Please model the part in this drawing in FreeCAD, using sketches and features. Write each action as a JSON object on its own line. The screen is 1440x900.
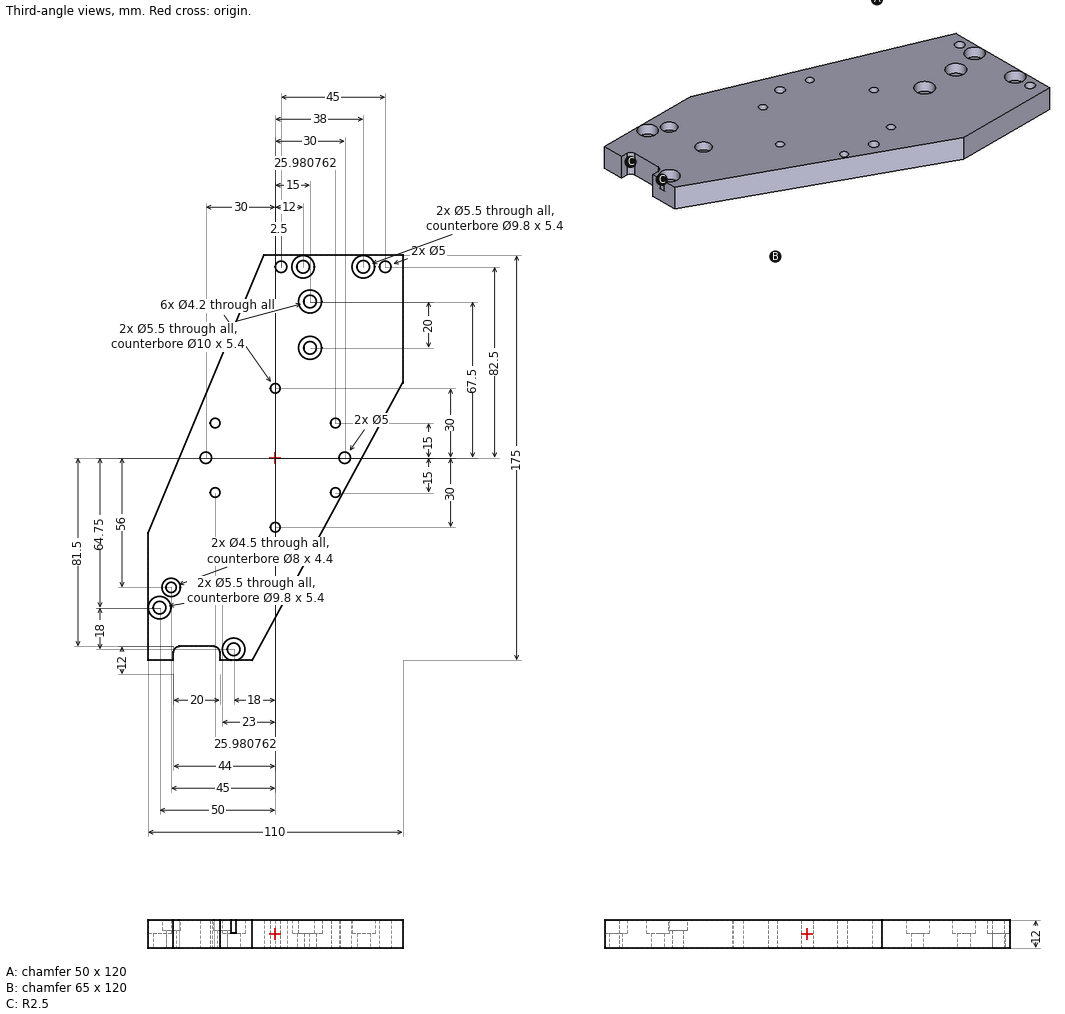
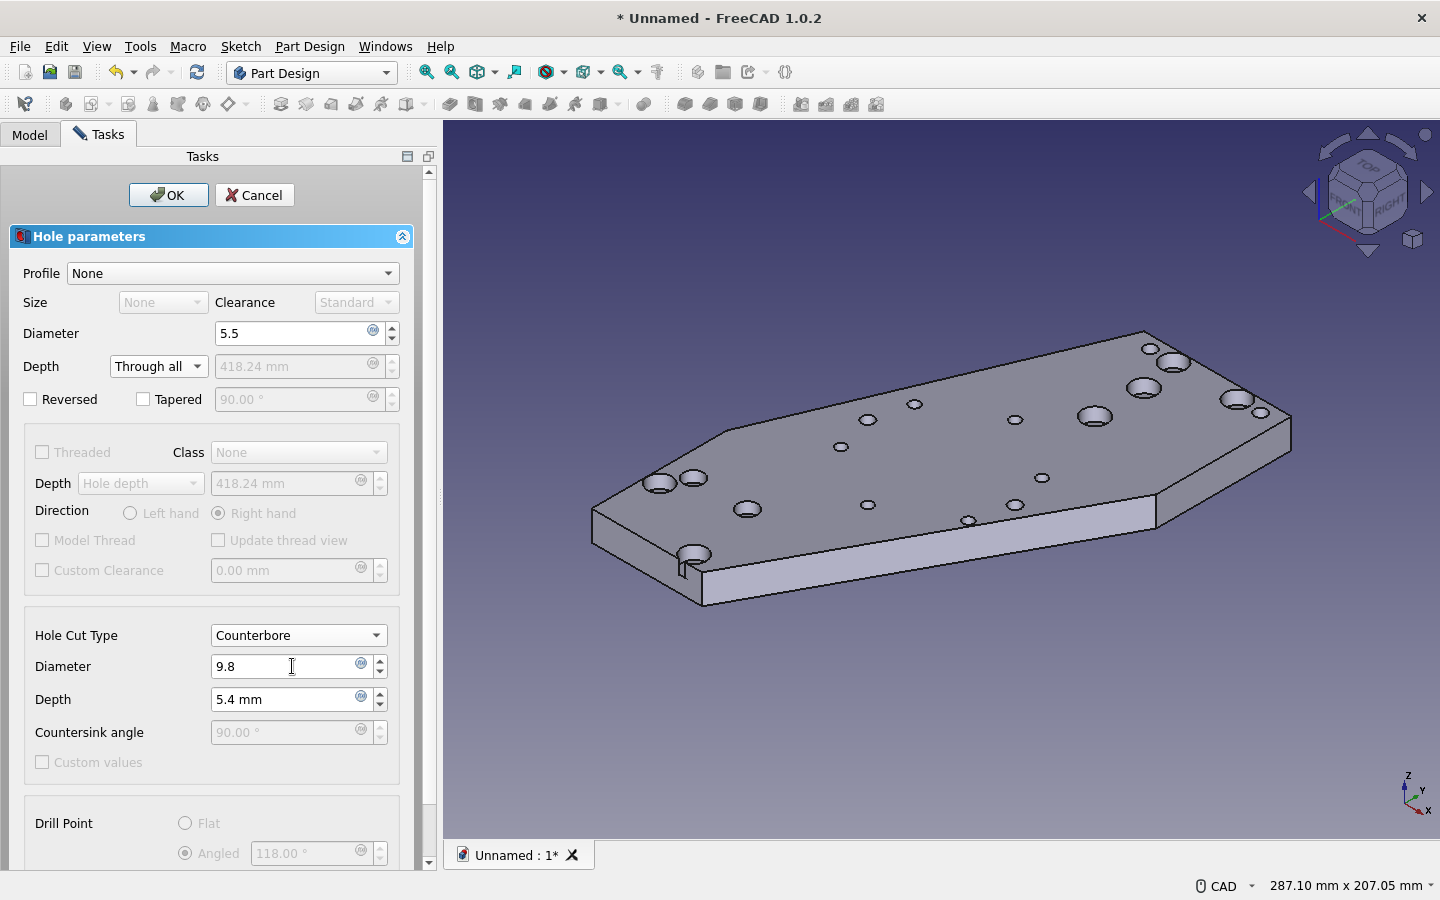
{"action": "left_click", "coordinate": [169, 195]}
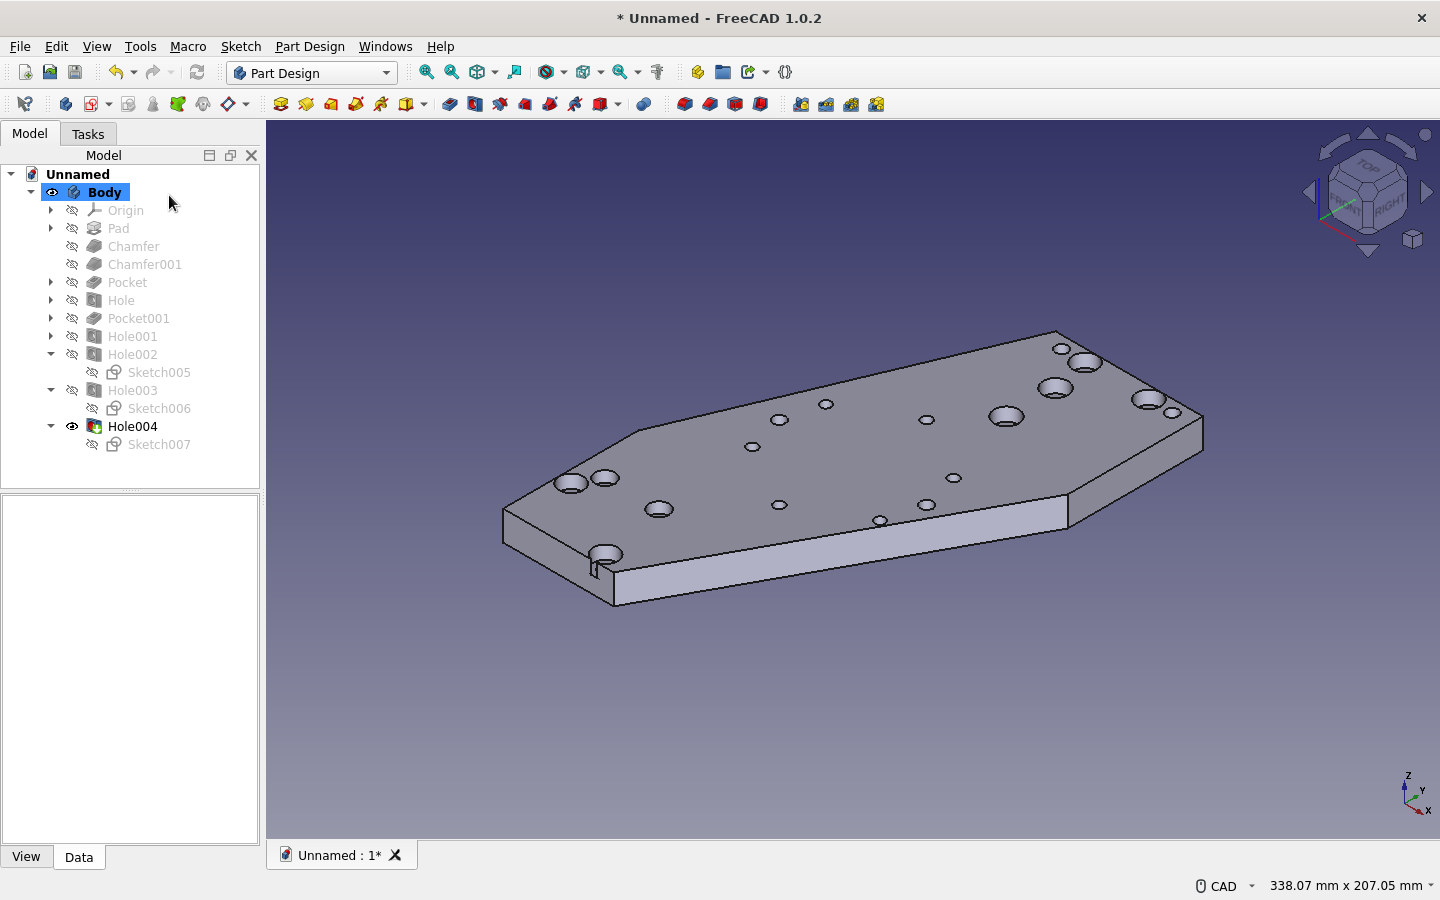
{"action": "left_click", "coordinate": [853, 461]}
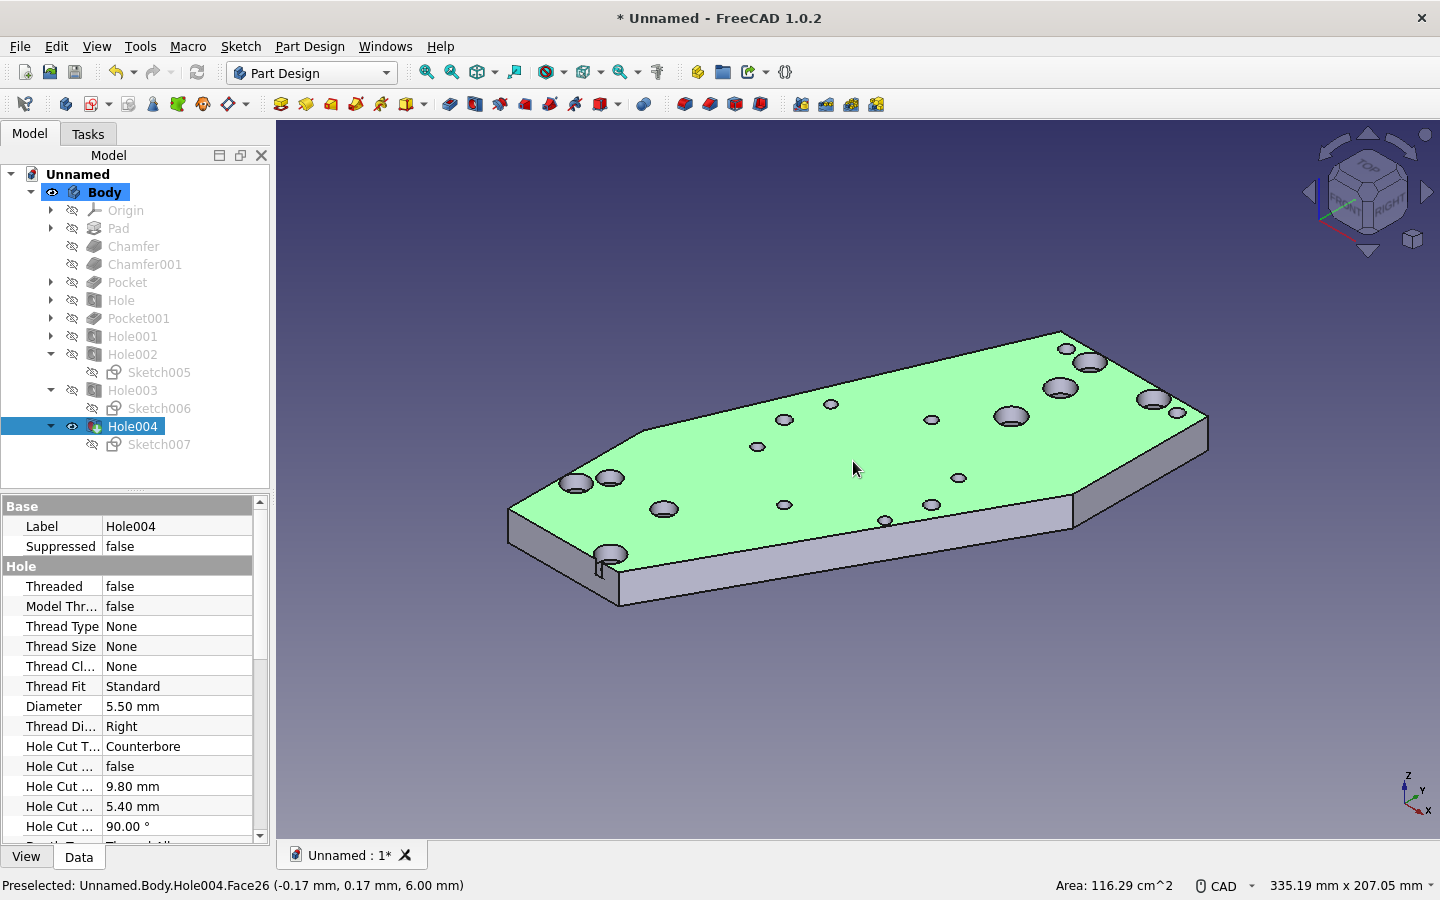
{"action": "left_click", "coordinate": [90, 104]}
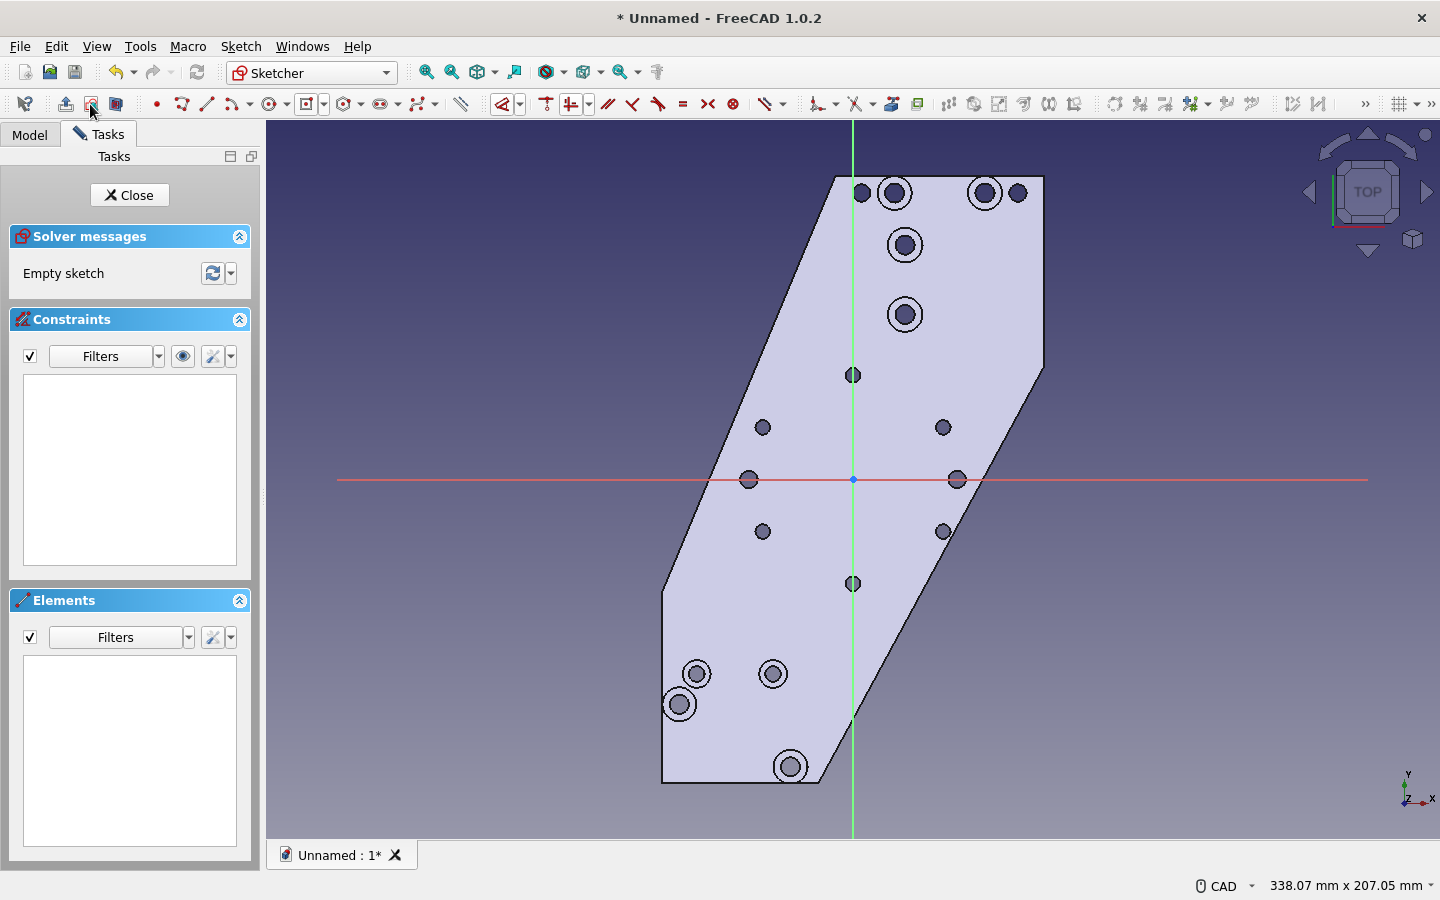
{"action": "scroll", "coordinate": [729, 811], "scroll_direction": "up", "scroll_amount": 11}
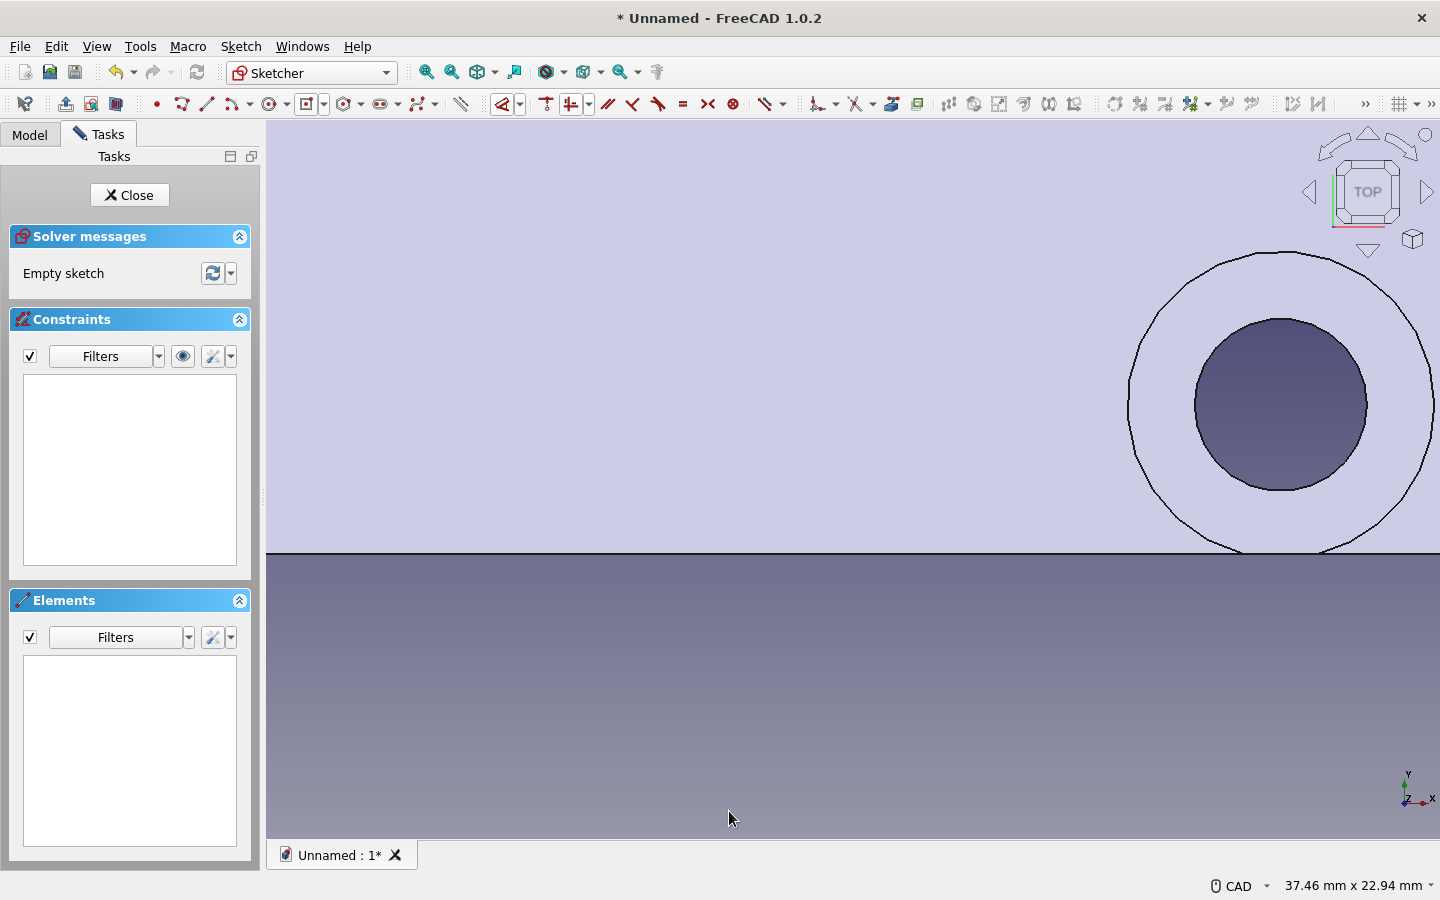
{"action": "key", "text": "g r"}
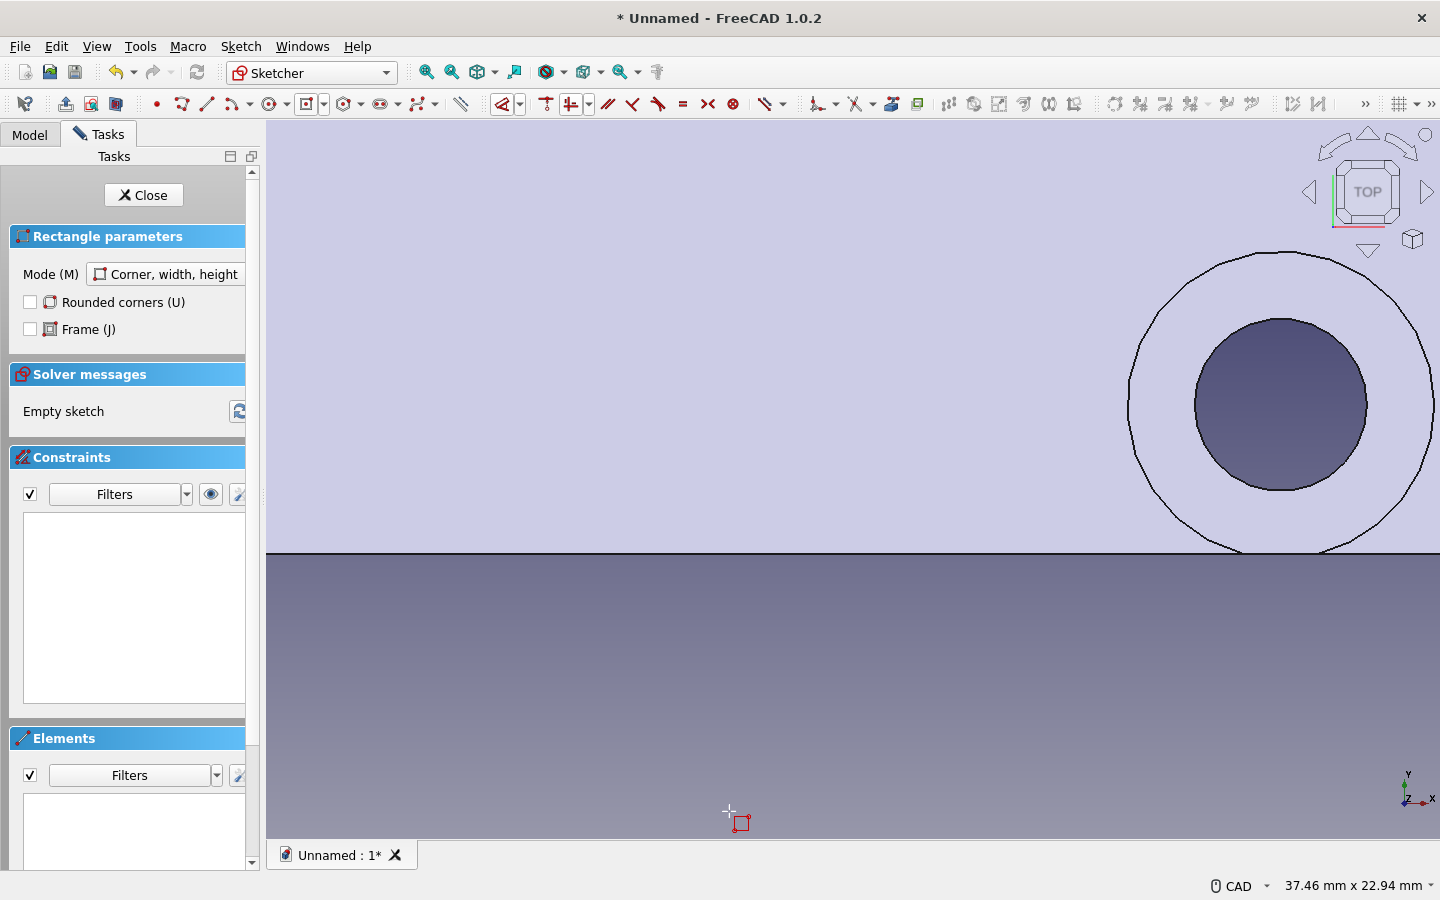
{"action": "left_click", "coordinate": [466, 366]}
{"action": "left_click", "coordinate": [1093, 742]}
{"action": "key", "text": "Escape"}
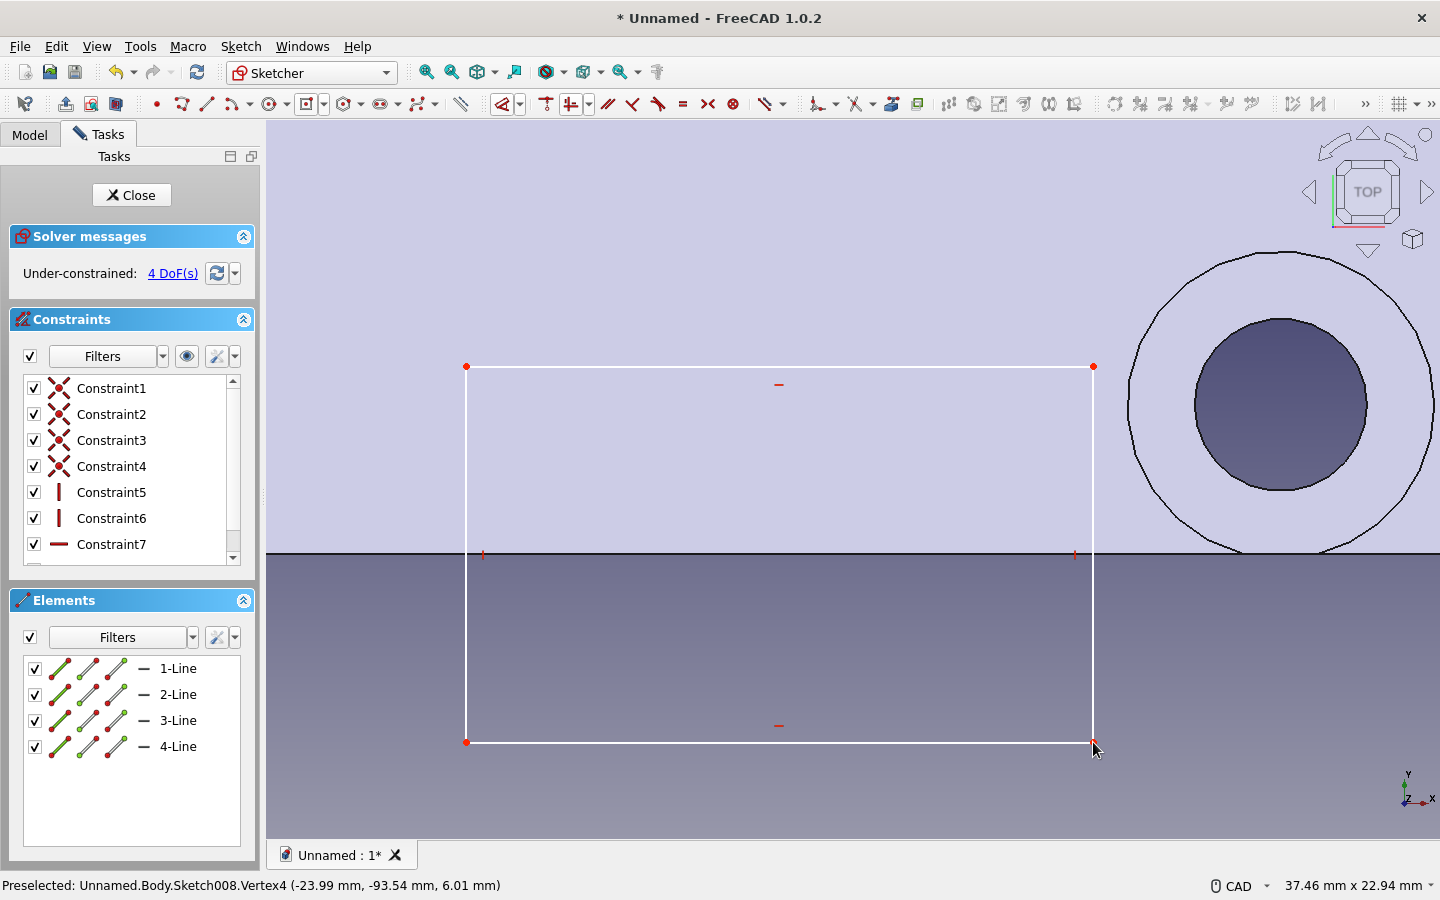
{"action": "left_click", "coordinate": [466, 480]}